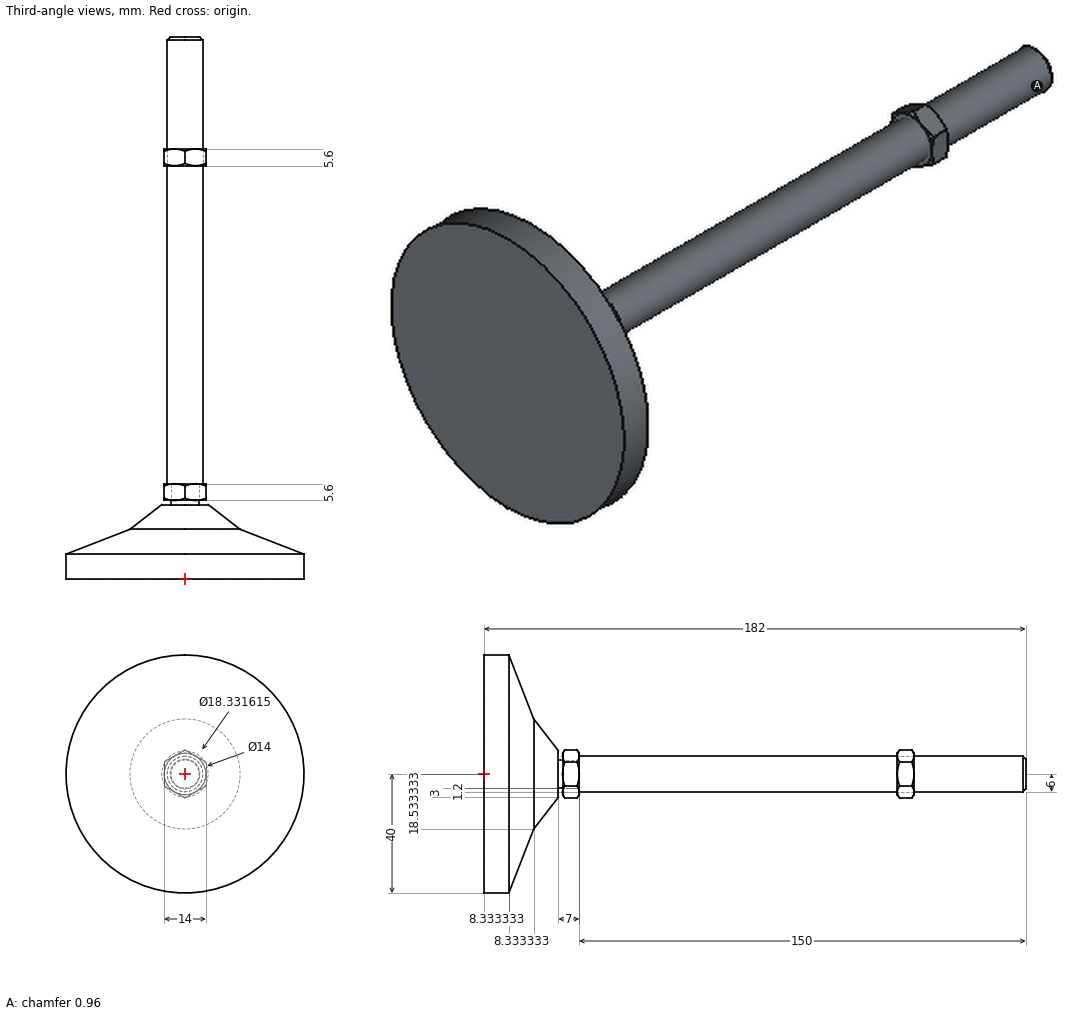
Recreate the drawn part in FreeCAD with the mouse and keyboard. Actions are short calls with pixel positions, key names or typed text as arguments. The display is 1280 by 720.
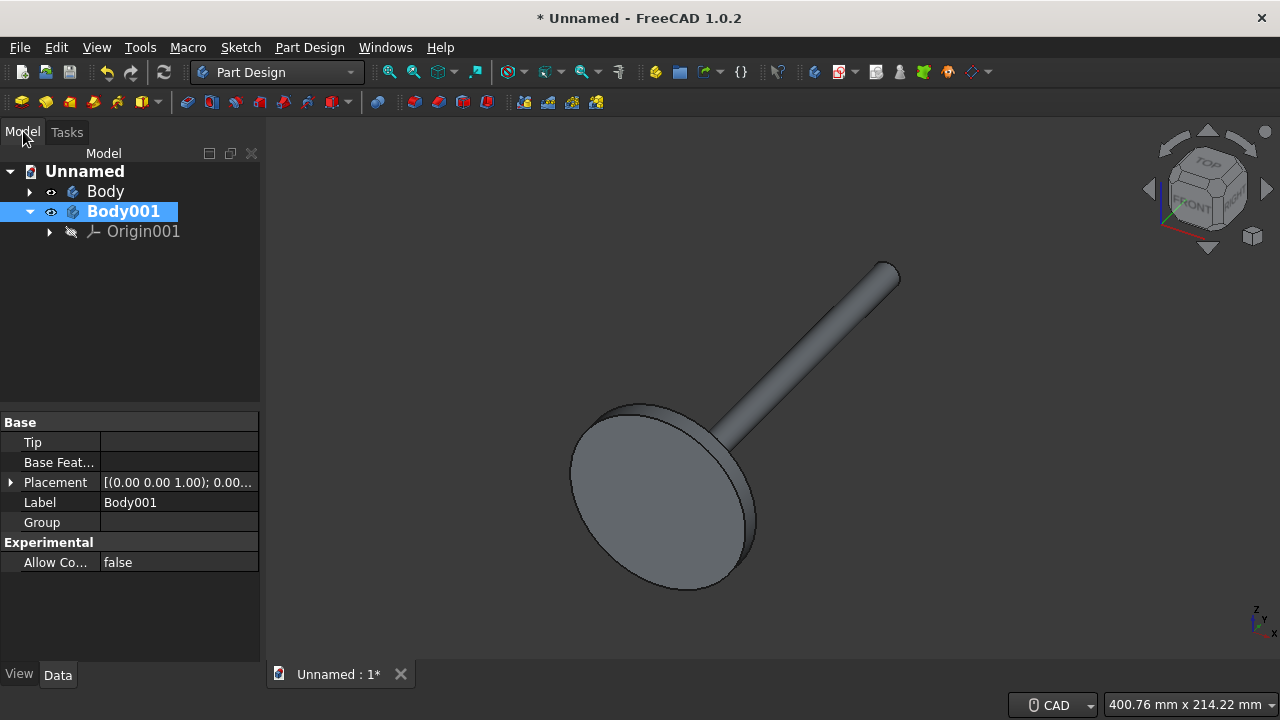
click(50, 232)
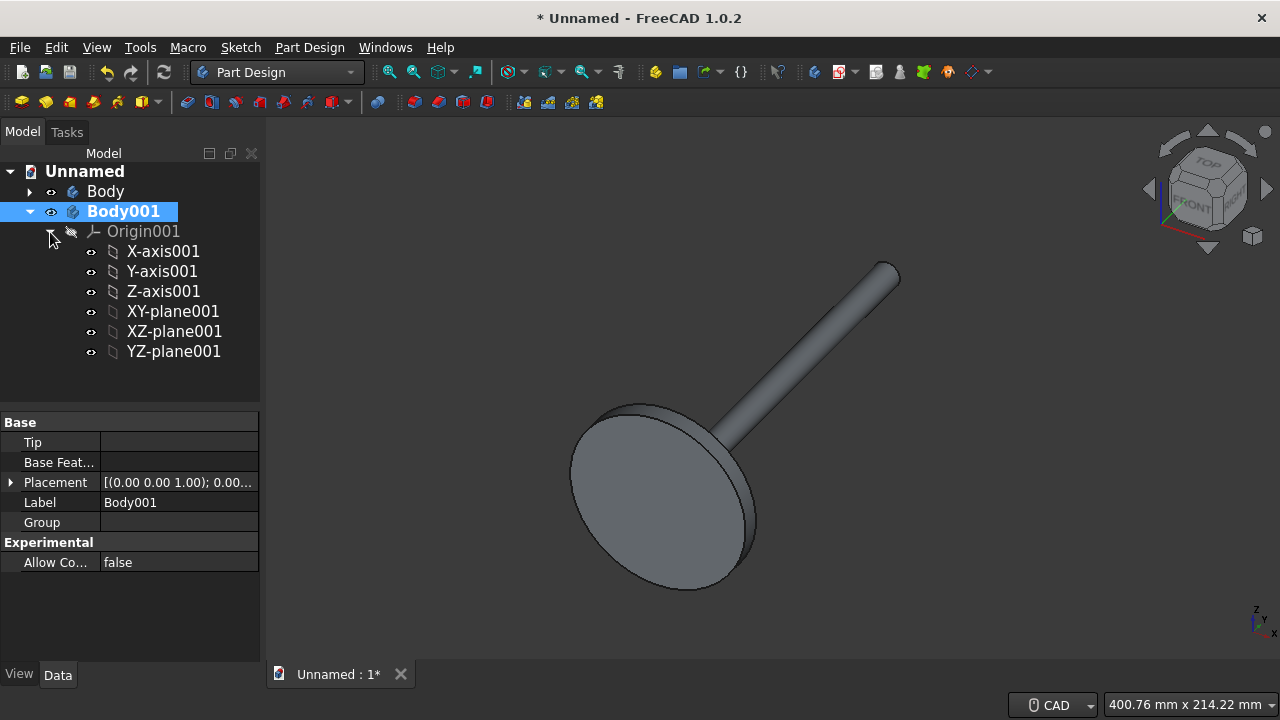
click(136, 332)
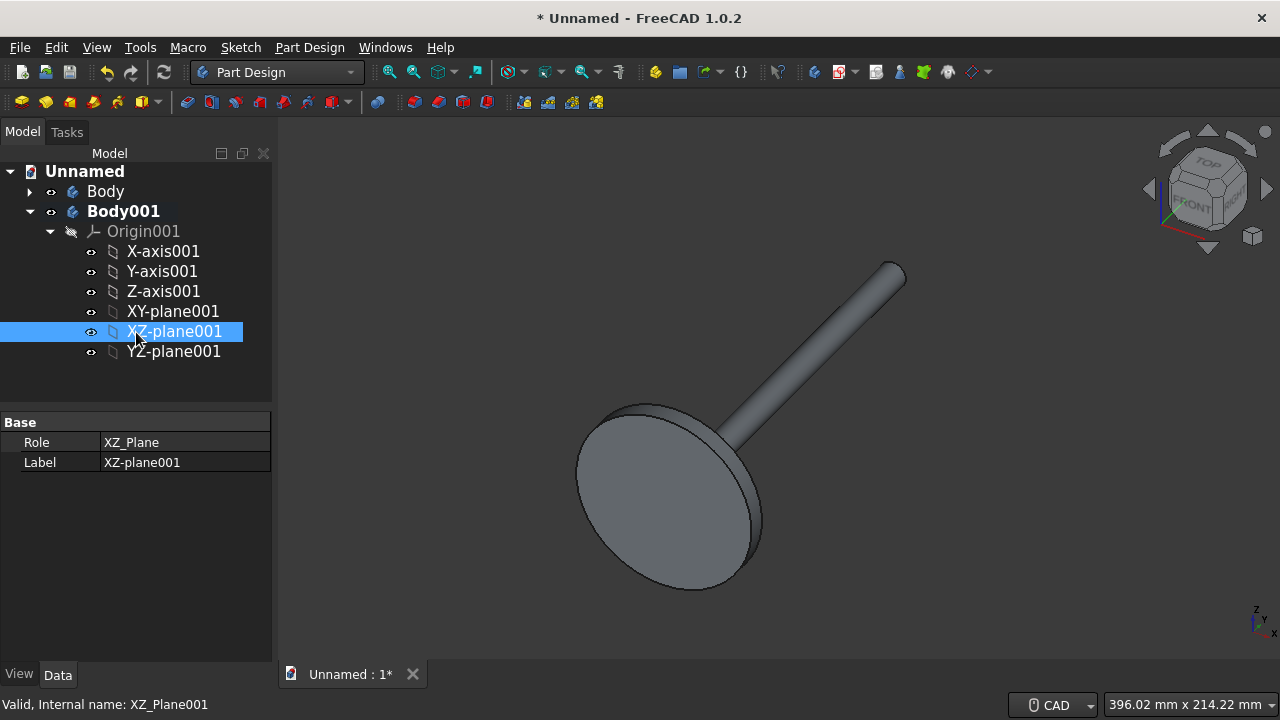
click(972, 72)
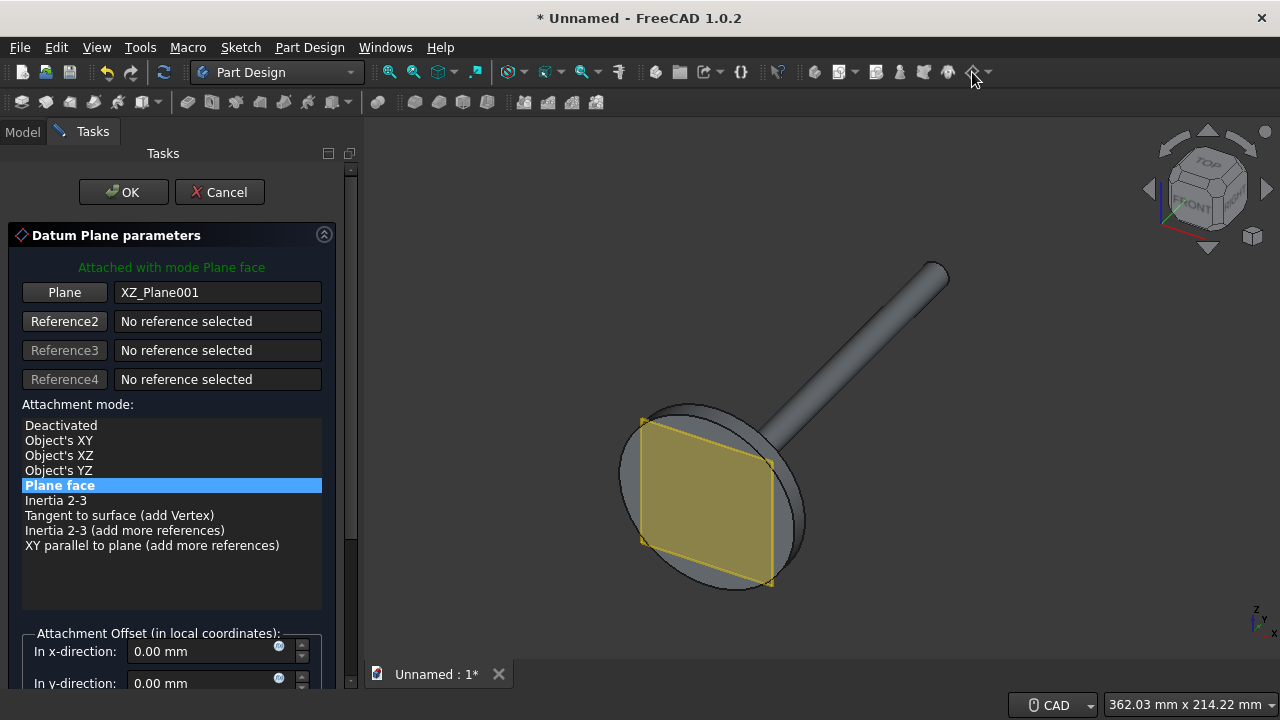
scroll(351, 426, down, 2)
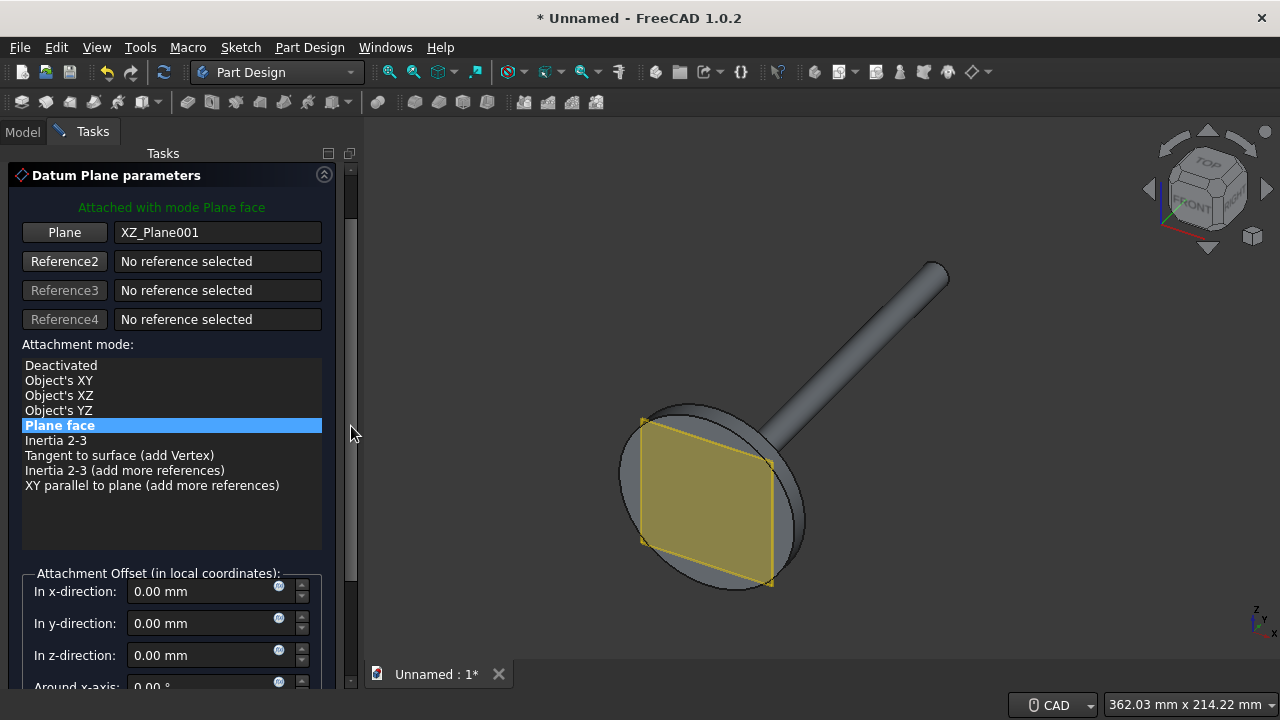
triple_click(210, 595)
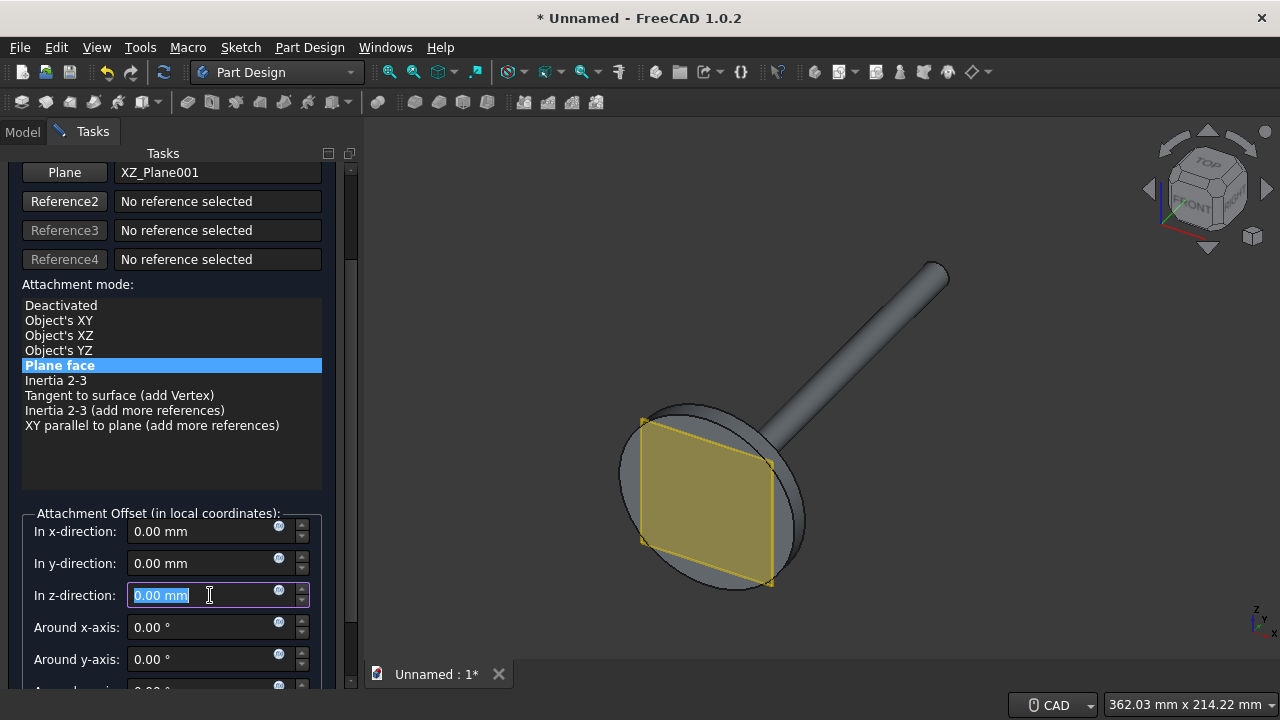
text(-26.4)
key(Tab)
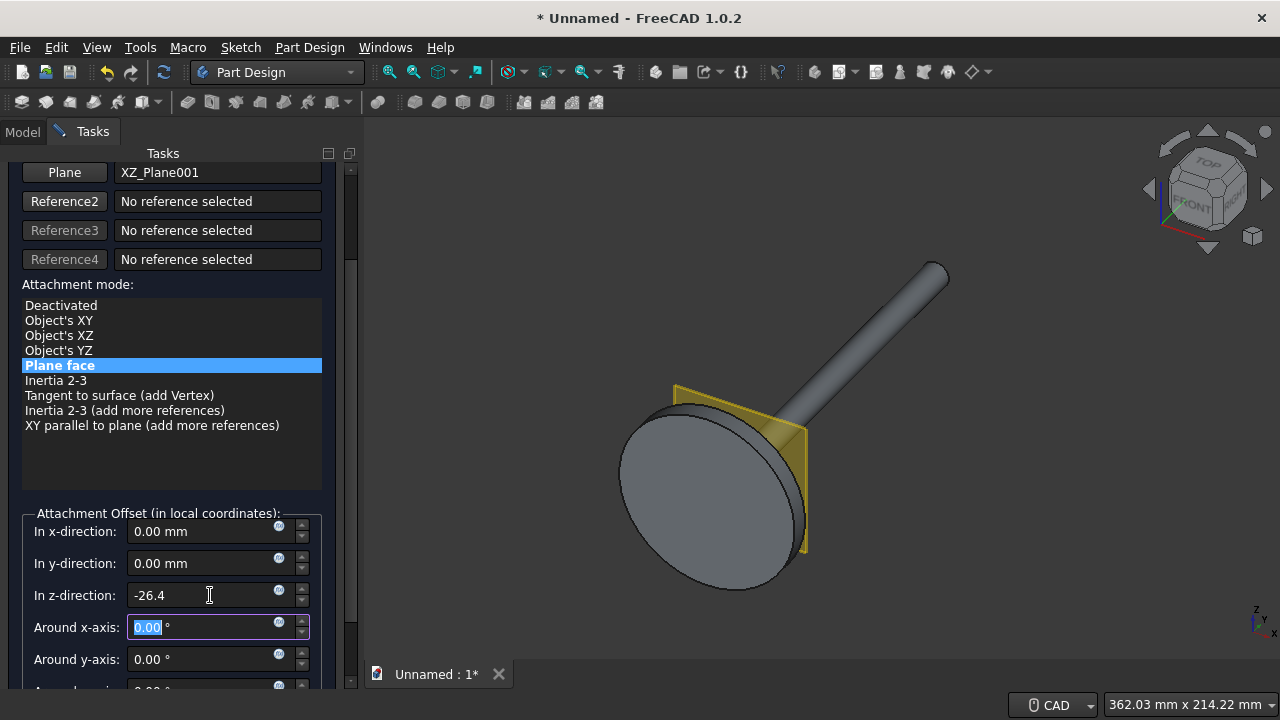
scroll(351, 426, up, 3)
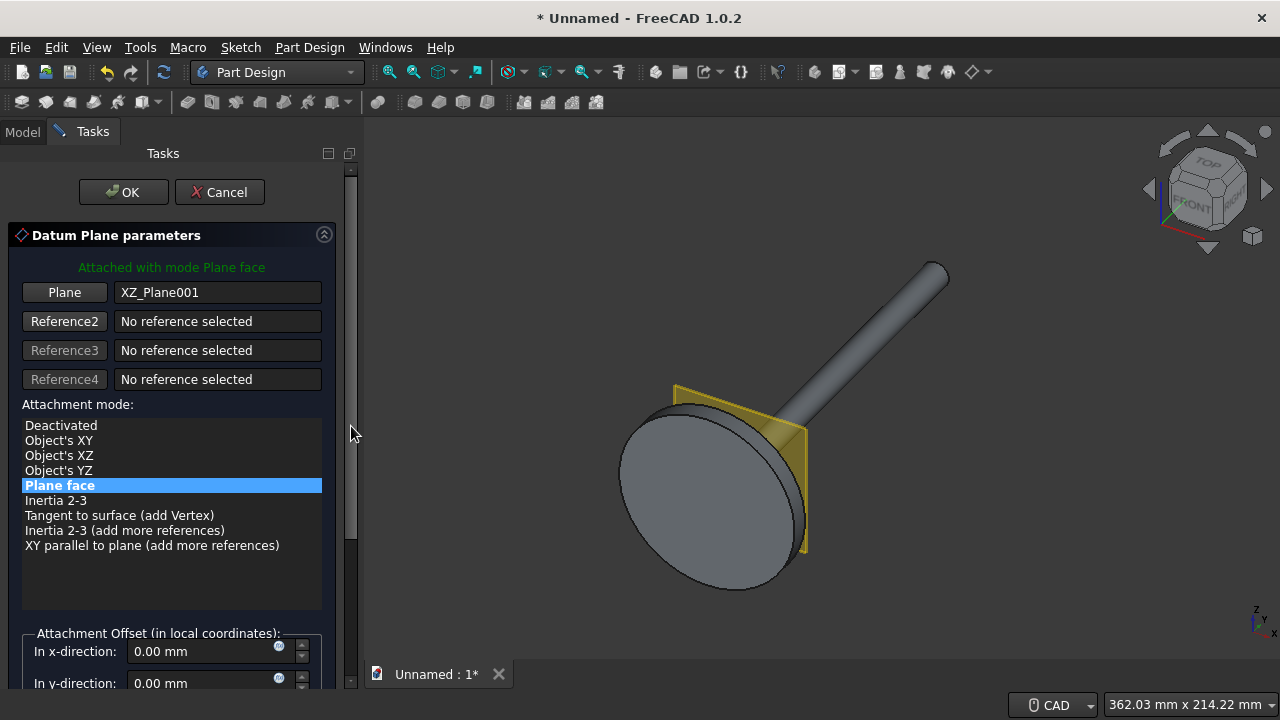
click(124, 192)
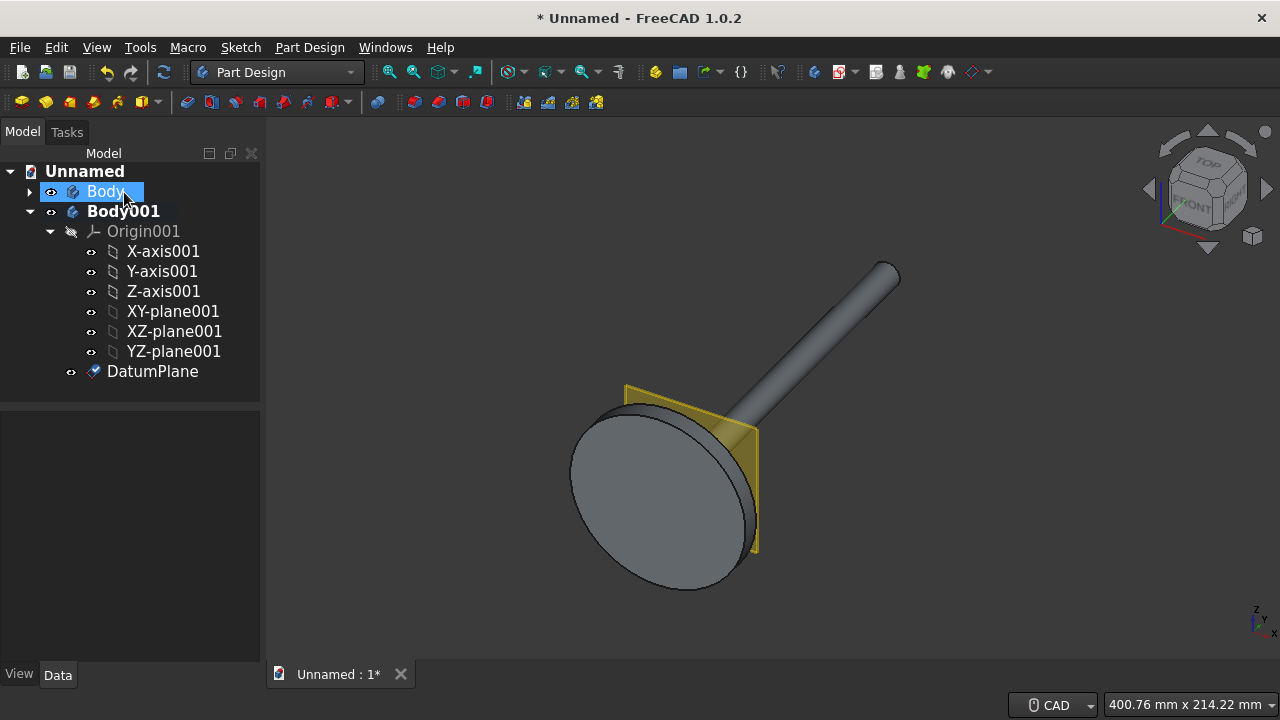
click(116, 372)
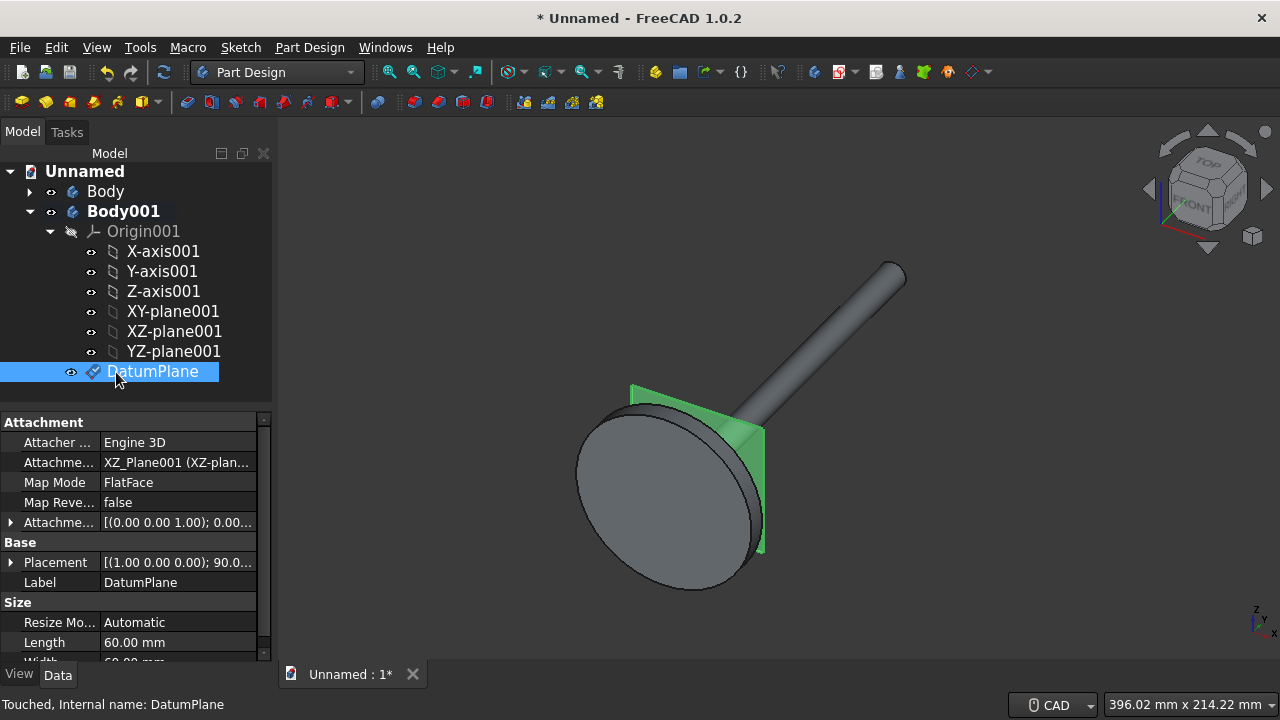
click(840, 72)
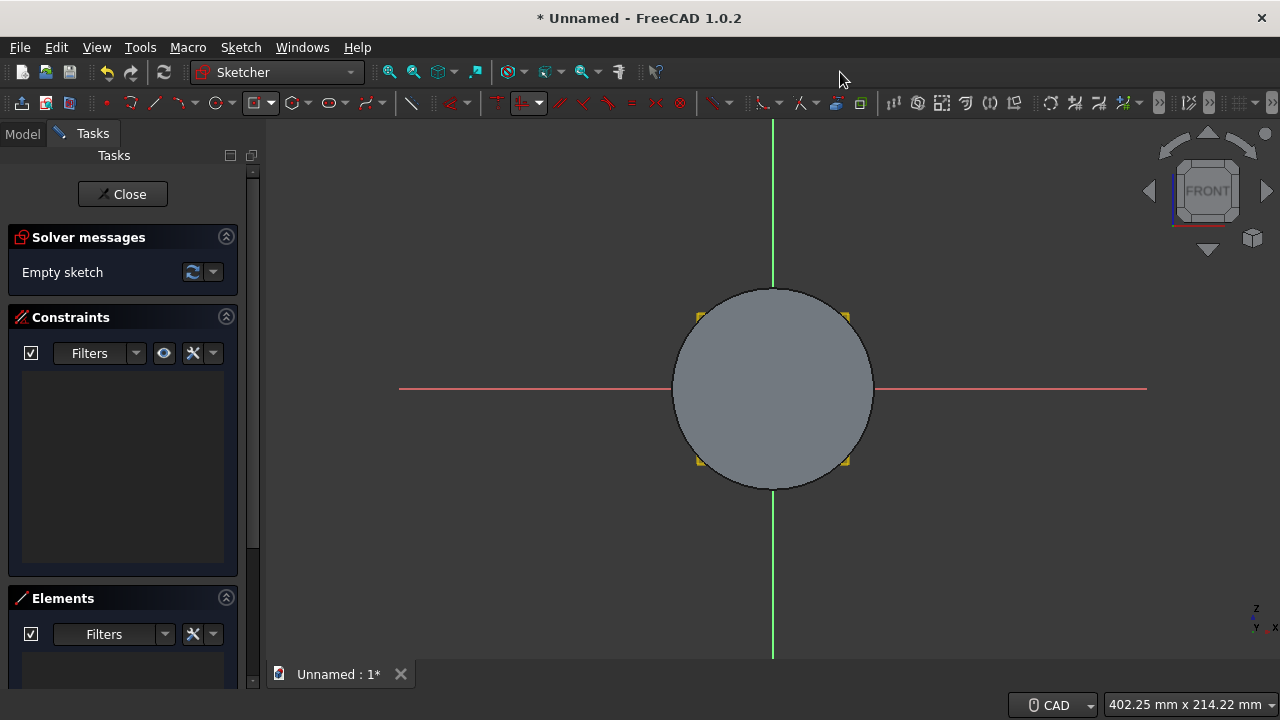
scroll(782, 389, up, 11)